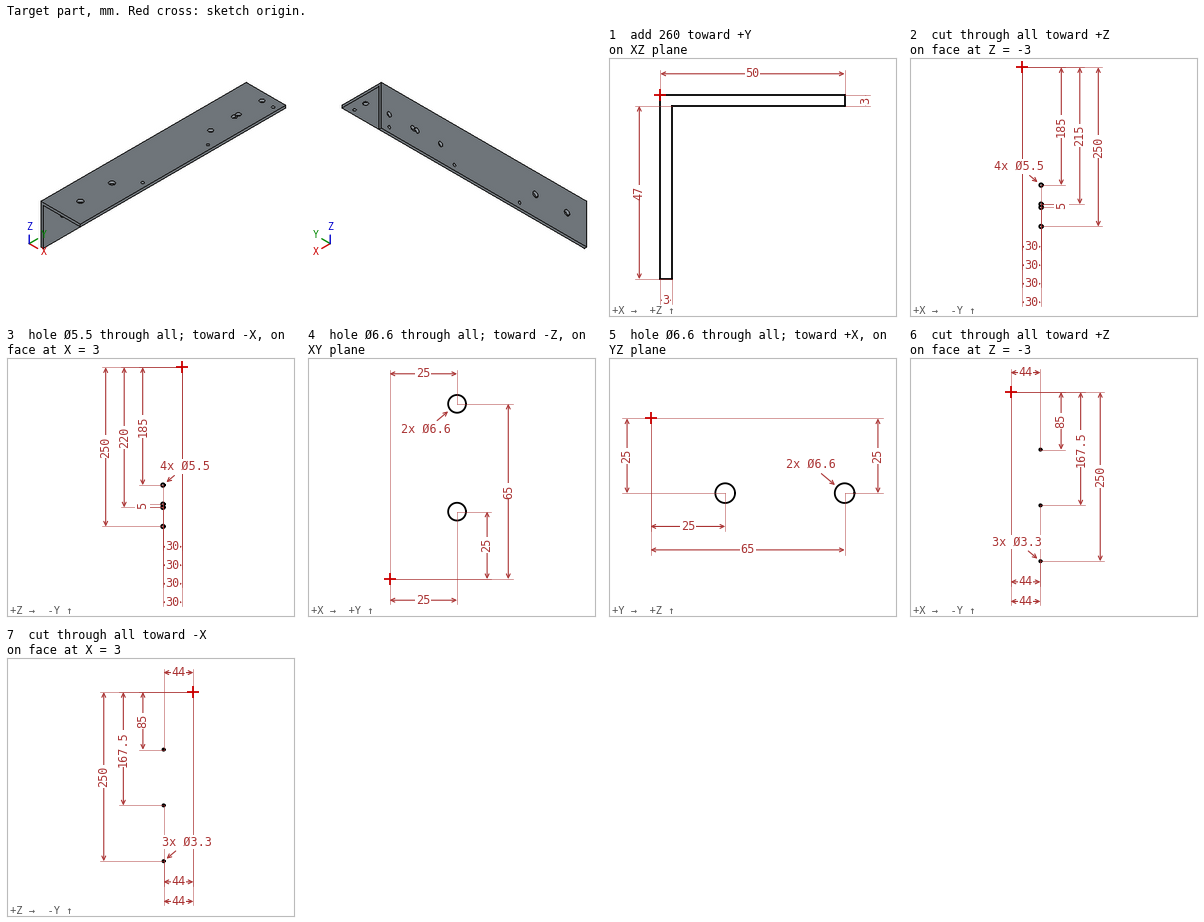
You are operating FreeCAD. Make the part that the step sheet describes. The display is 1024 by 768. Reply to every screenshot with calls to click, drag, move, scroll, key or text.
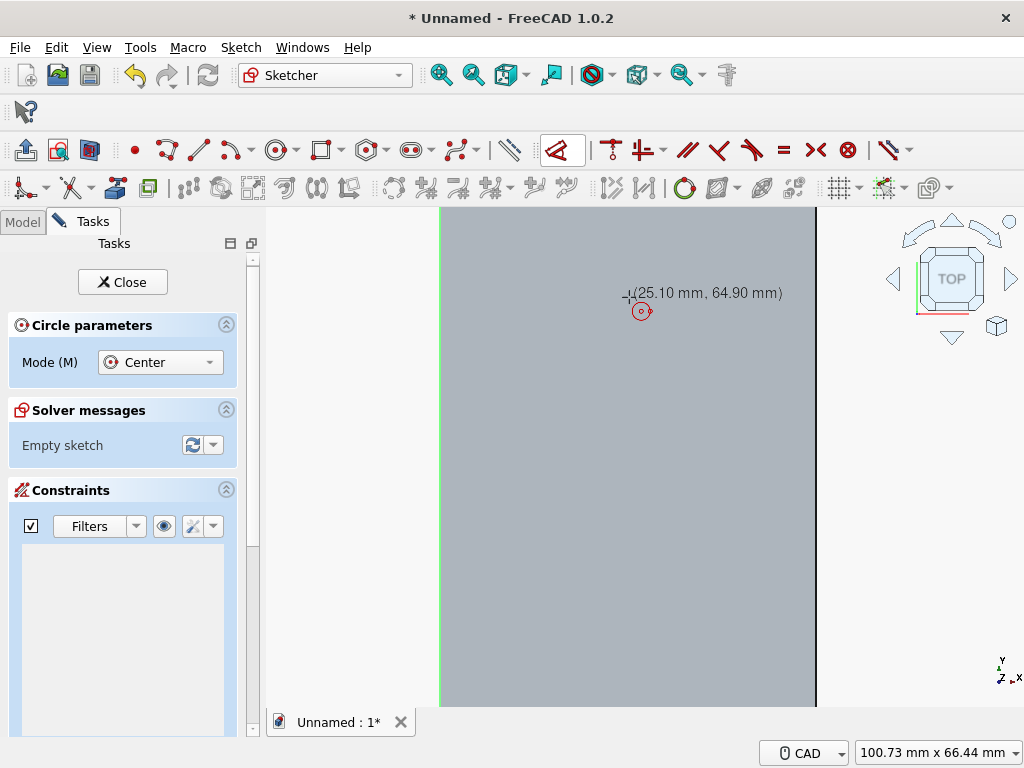
click(628, 298)
click(646, 280)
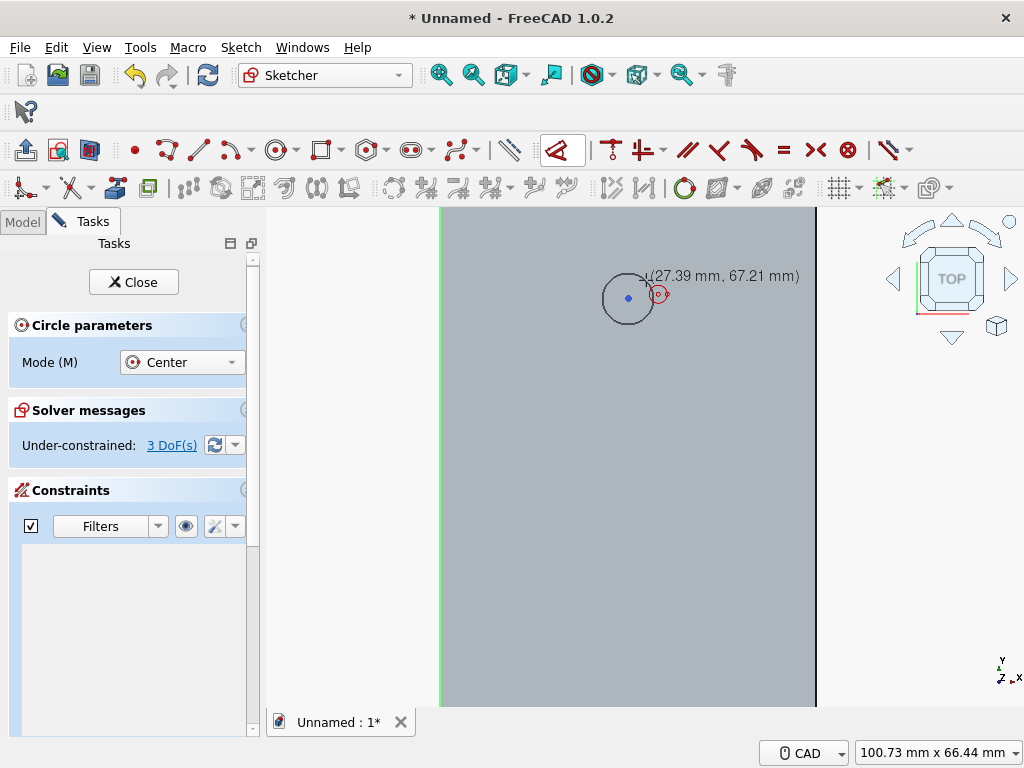
click(628, 599)
click(646, 581)
key(Escape)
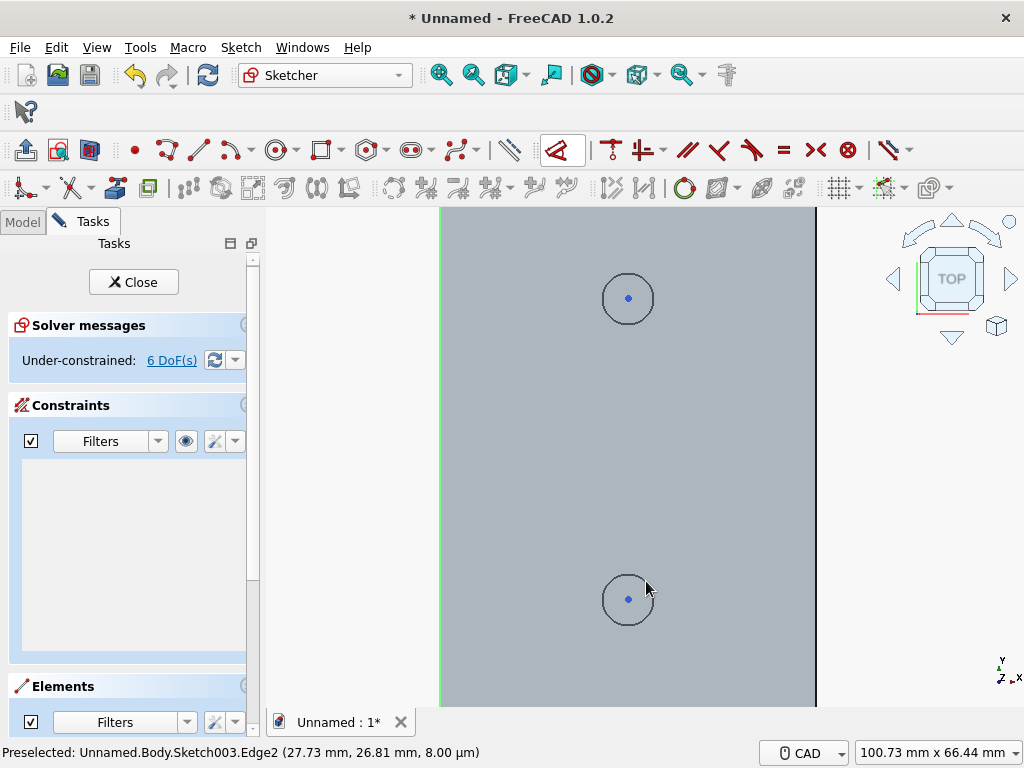
click(646, 281)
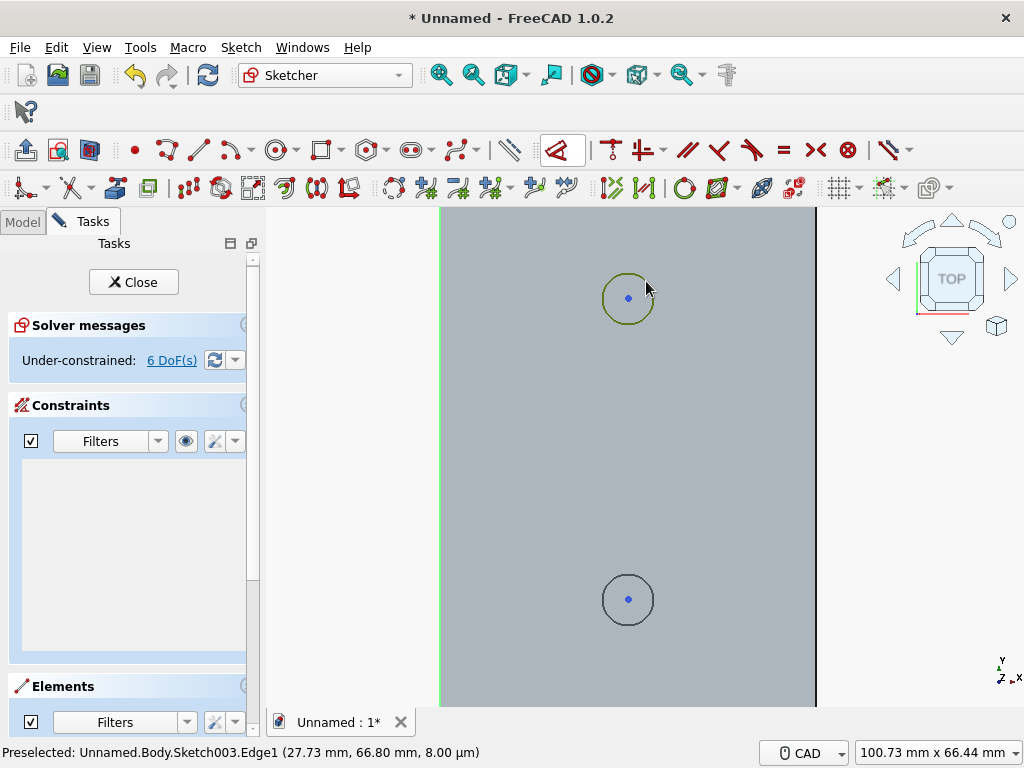
click(646, 582)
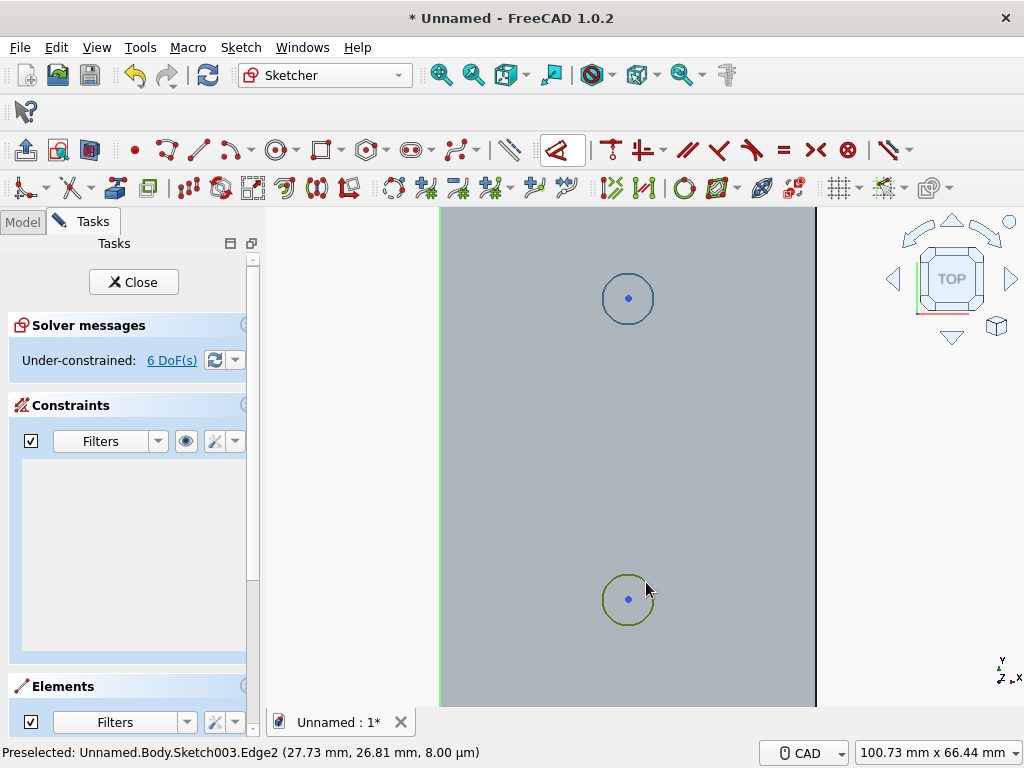
key(e)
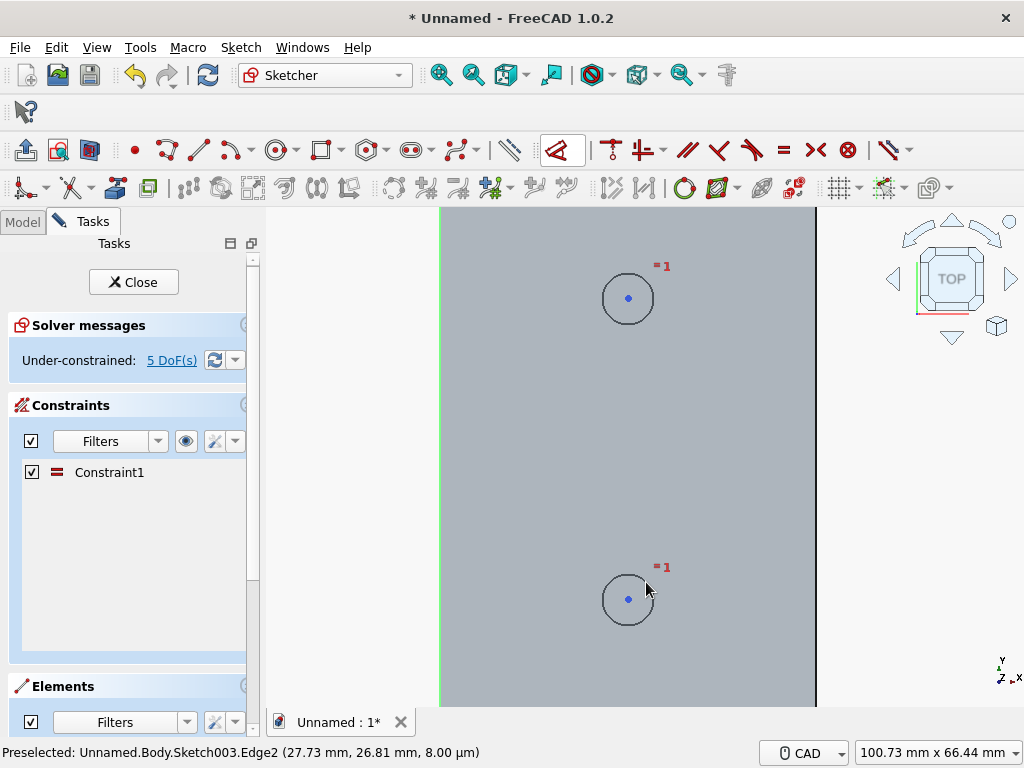
click(646, 281)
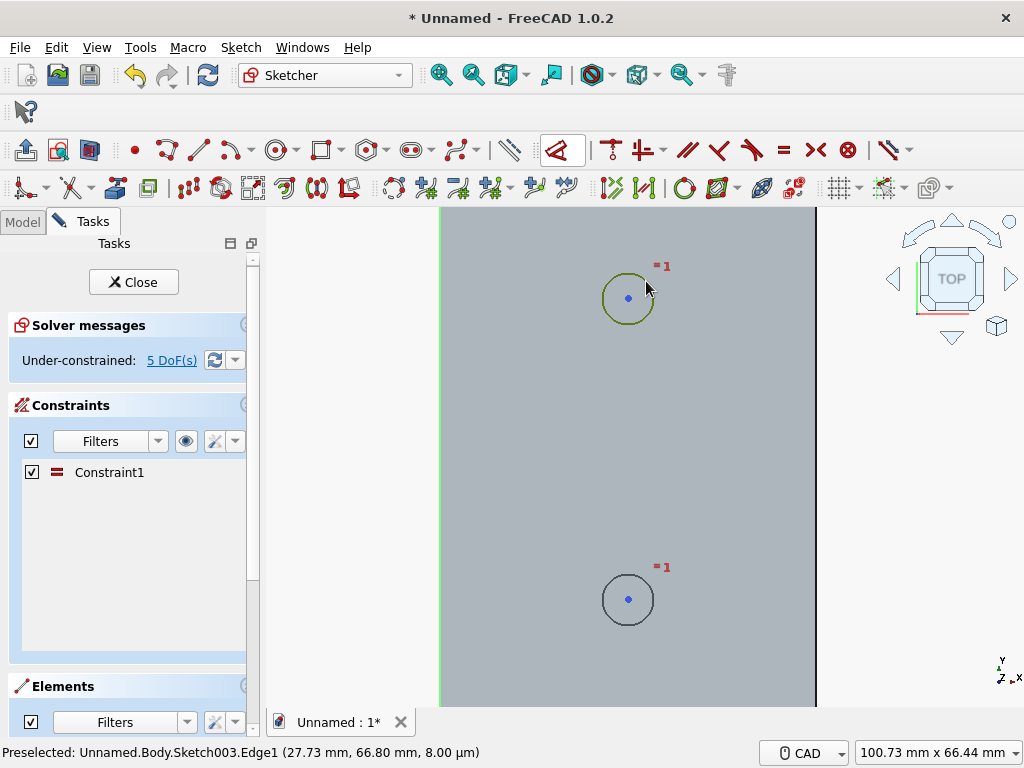
click(580, 150)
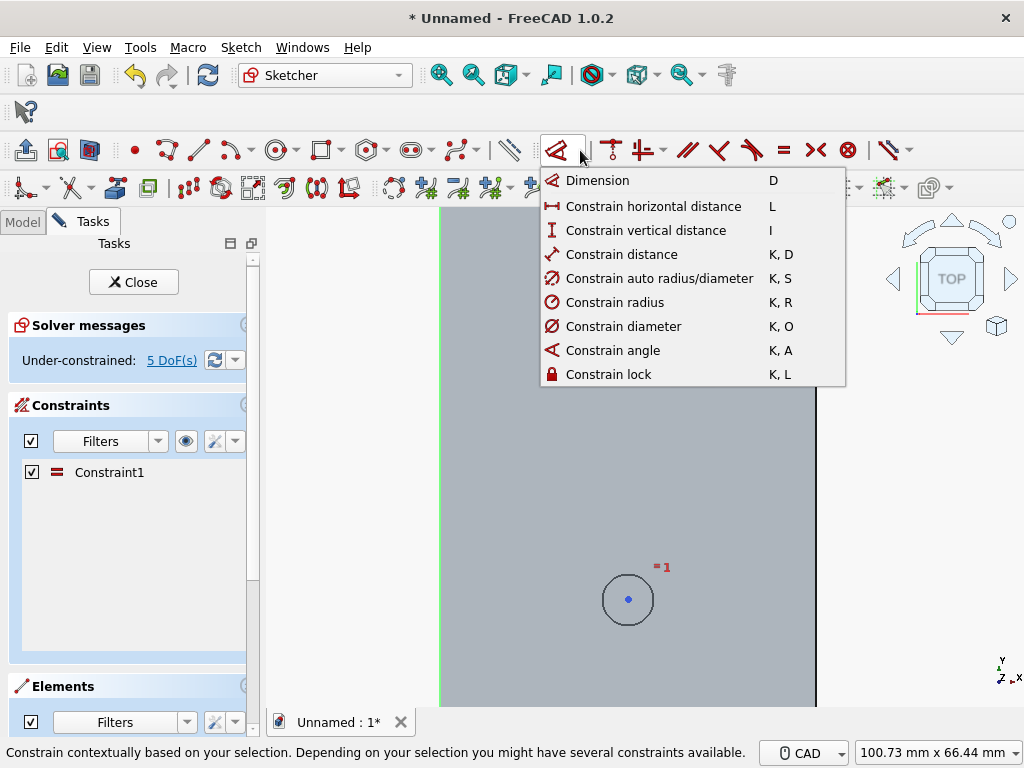
click(693, 326)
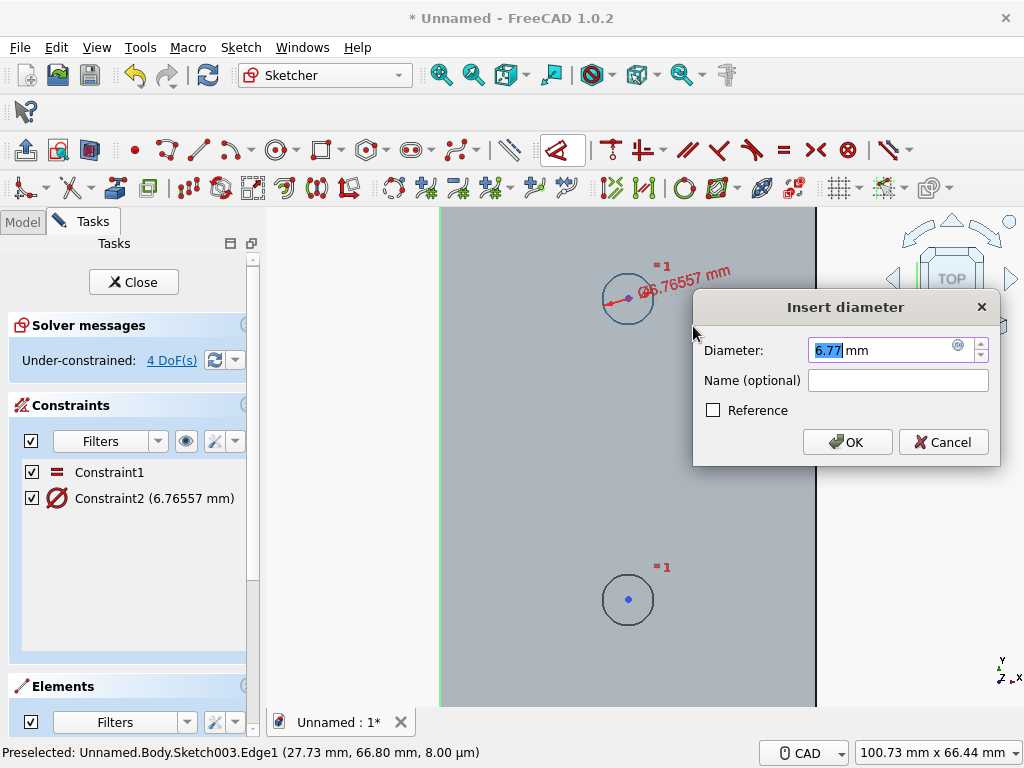
text(6.6)
key(Return)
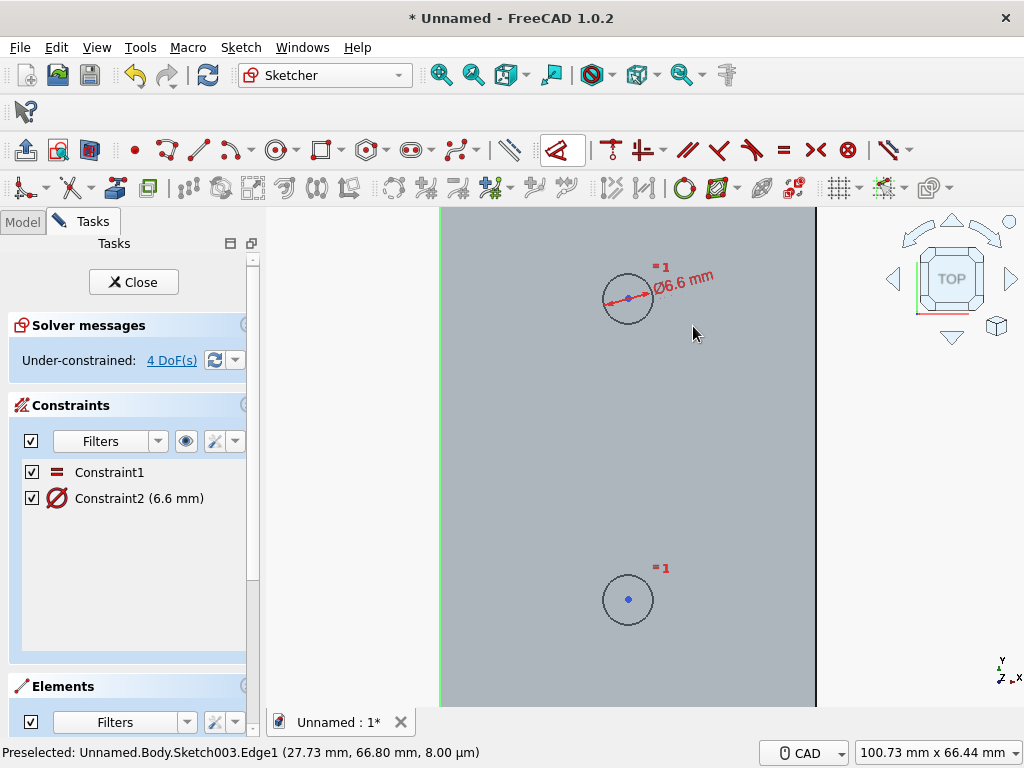
click(628, 299)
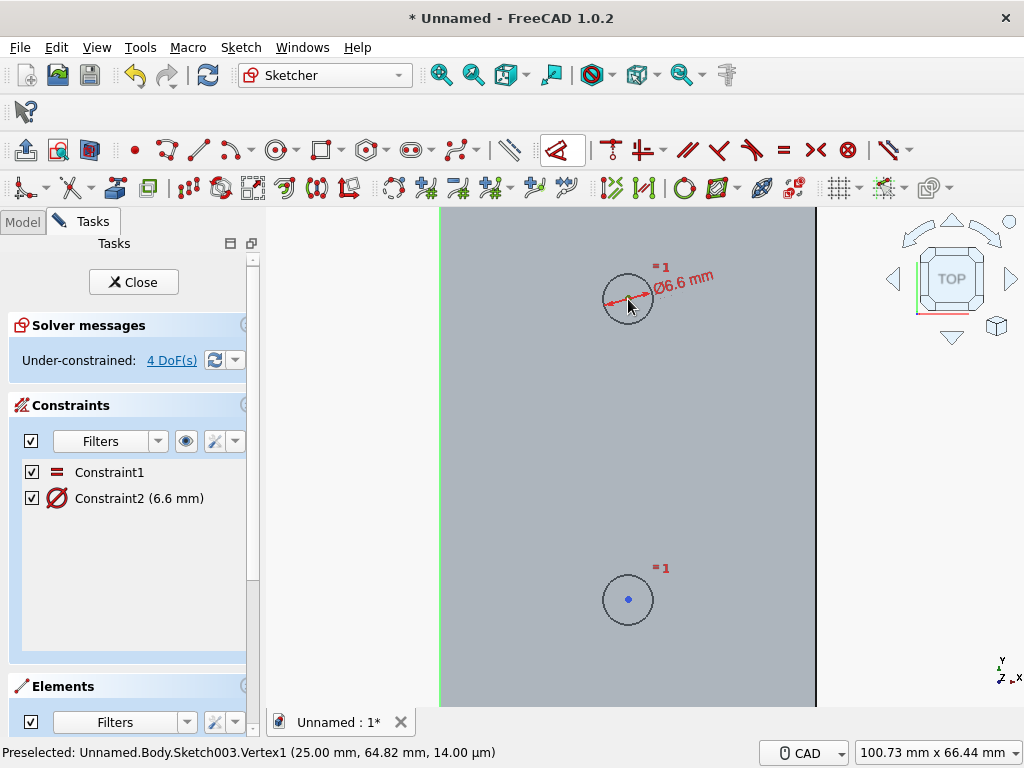
key(l)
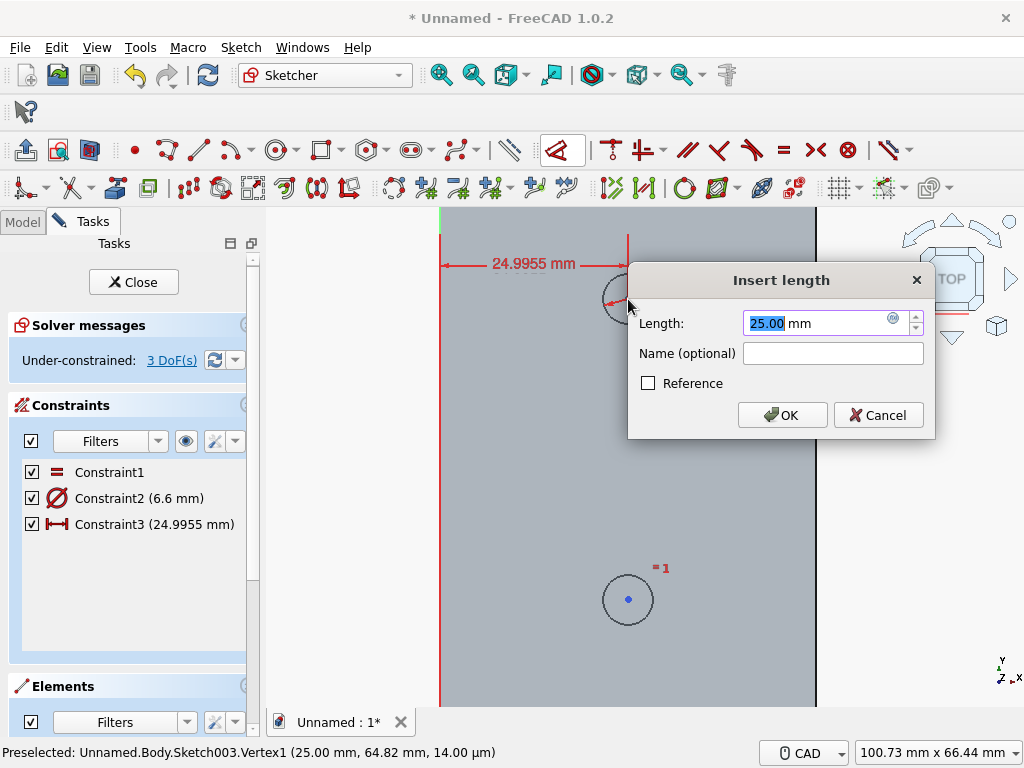
text(25)
key(Return)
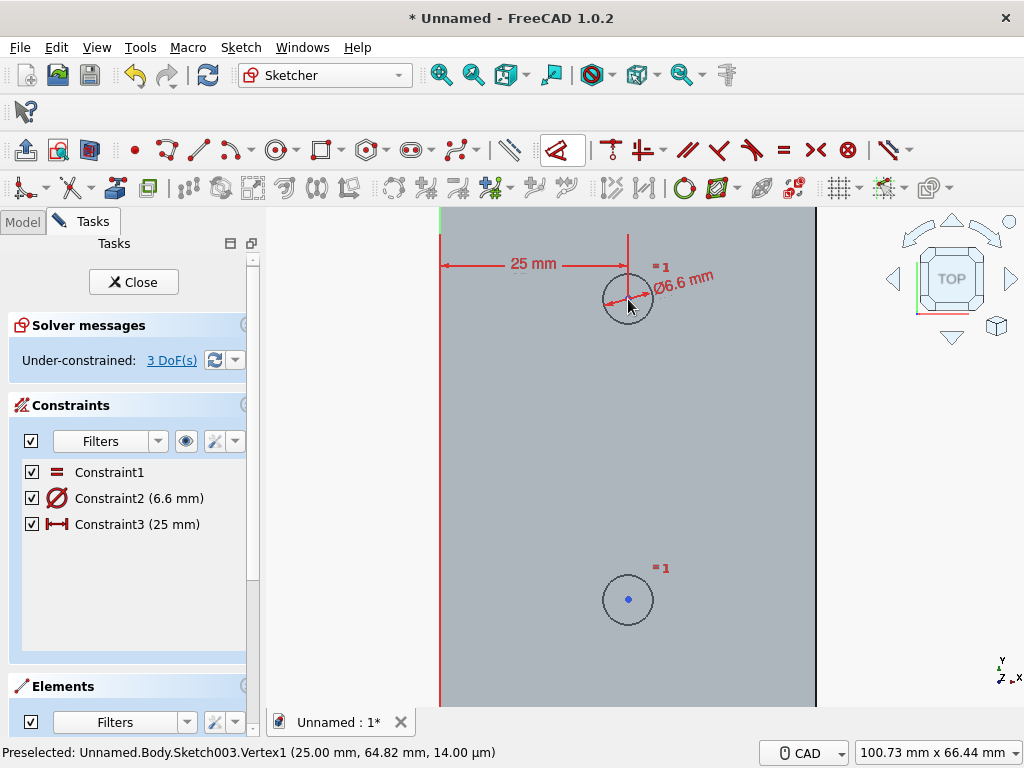
click(628, 299)